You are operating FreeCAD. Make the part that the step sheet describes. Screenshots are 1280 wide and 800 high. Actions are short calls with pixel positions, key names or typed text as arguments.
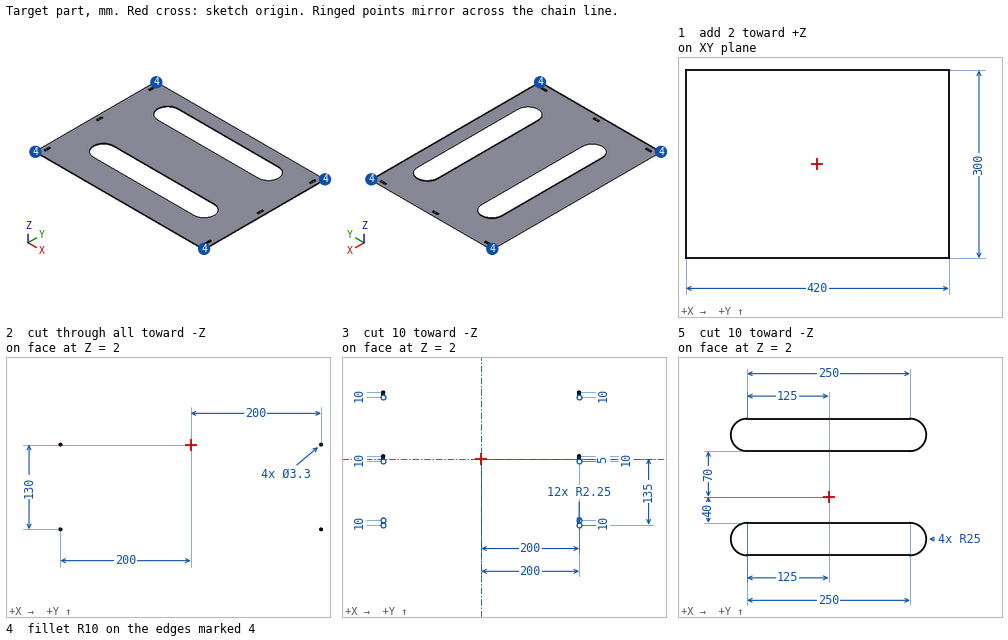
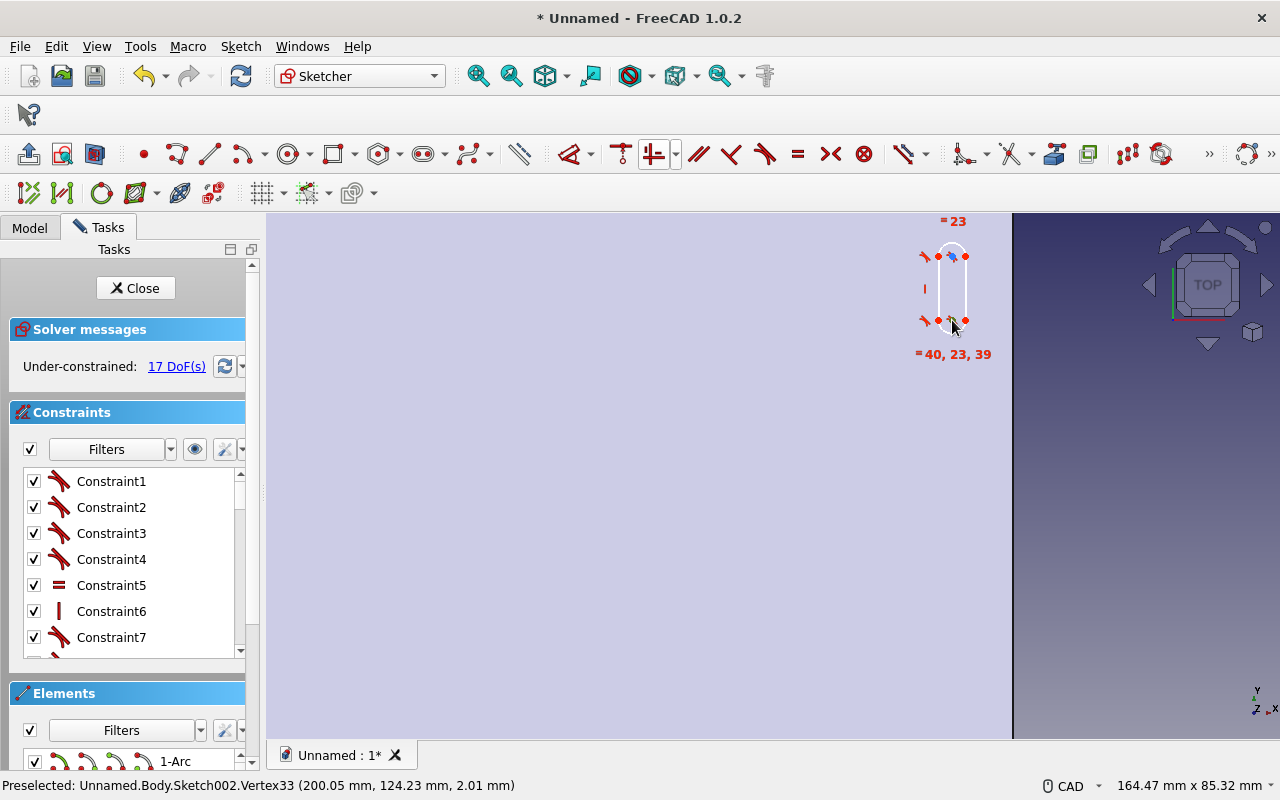
scroll(954, 322, down, 8)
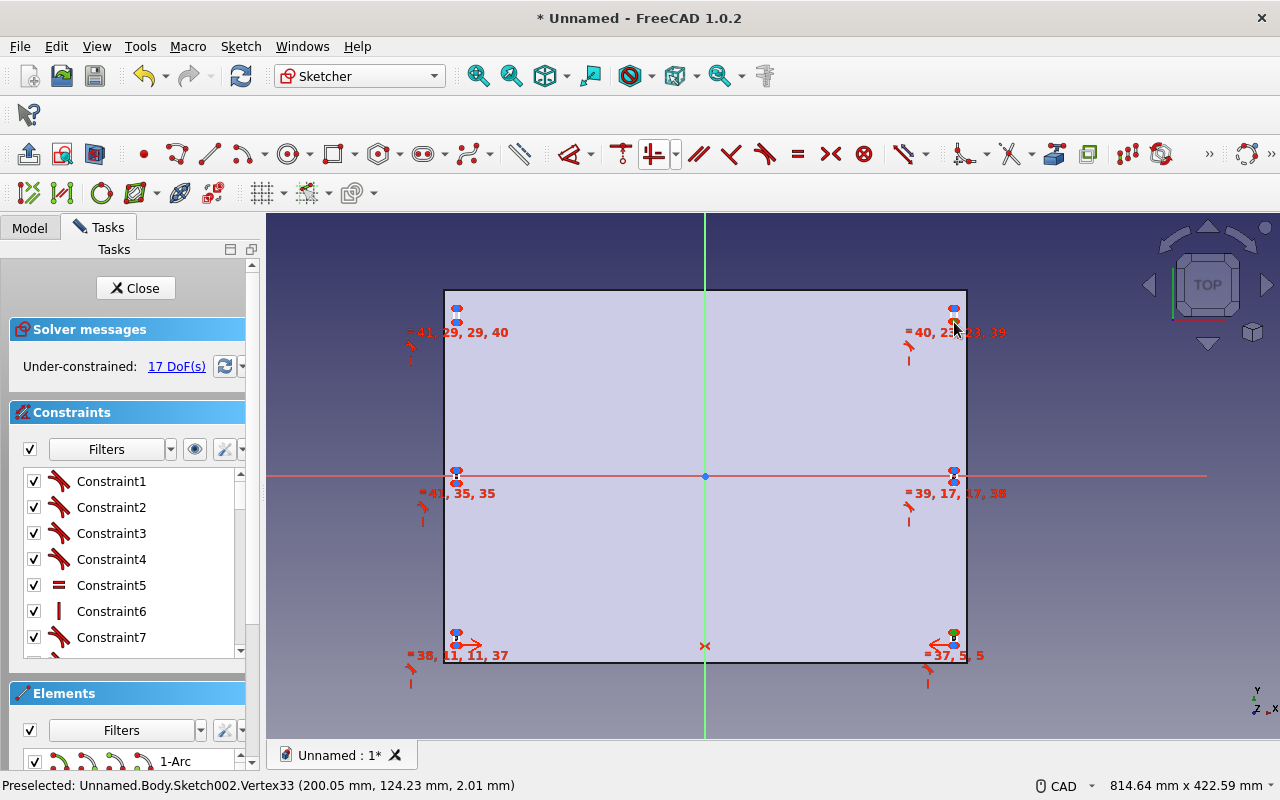
click(353, 476)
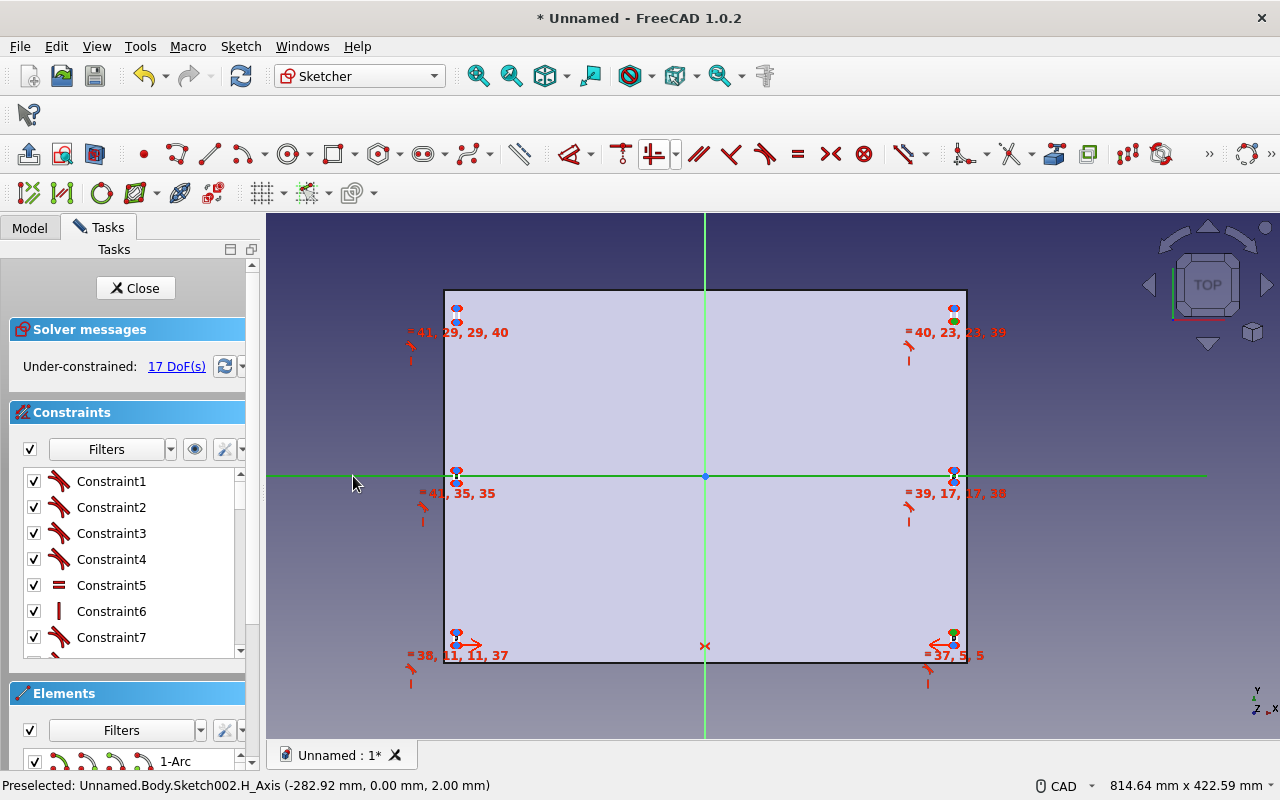
click(831, 154)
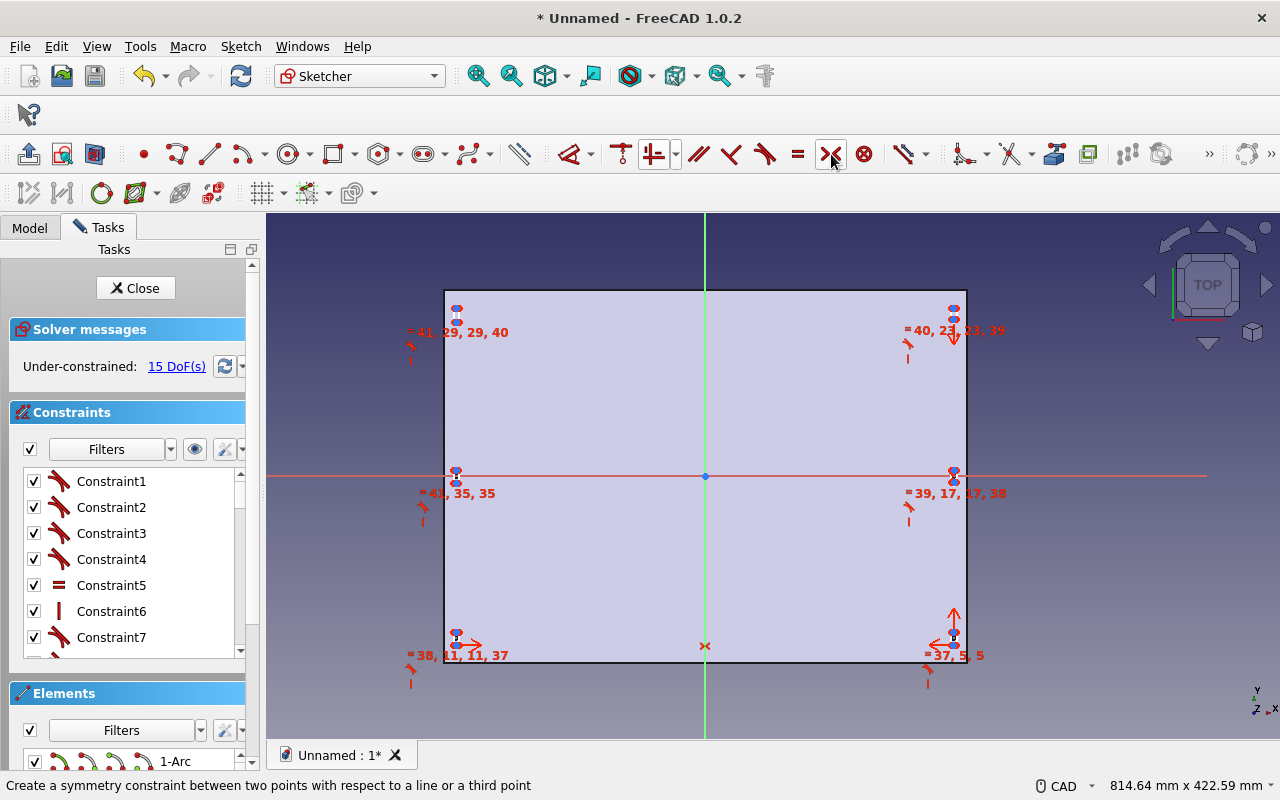
scroll(456, 633, up, 8)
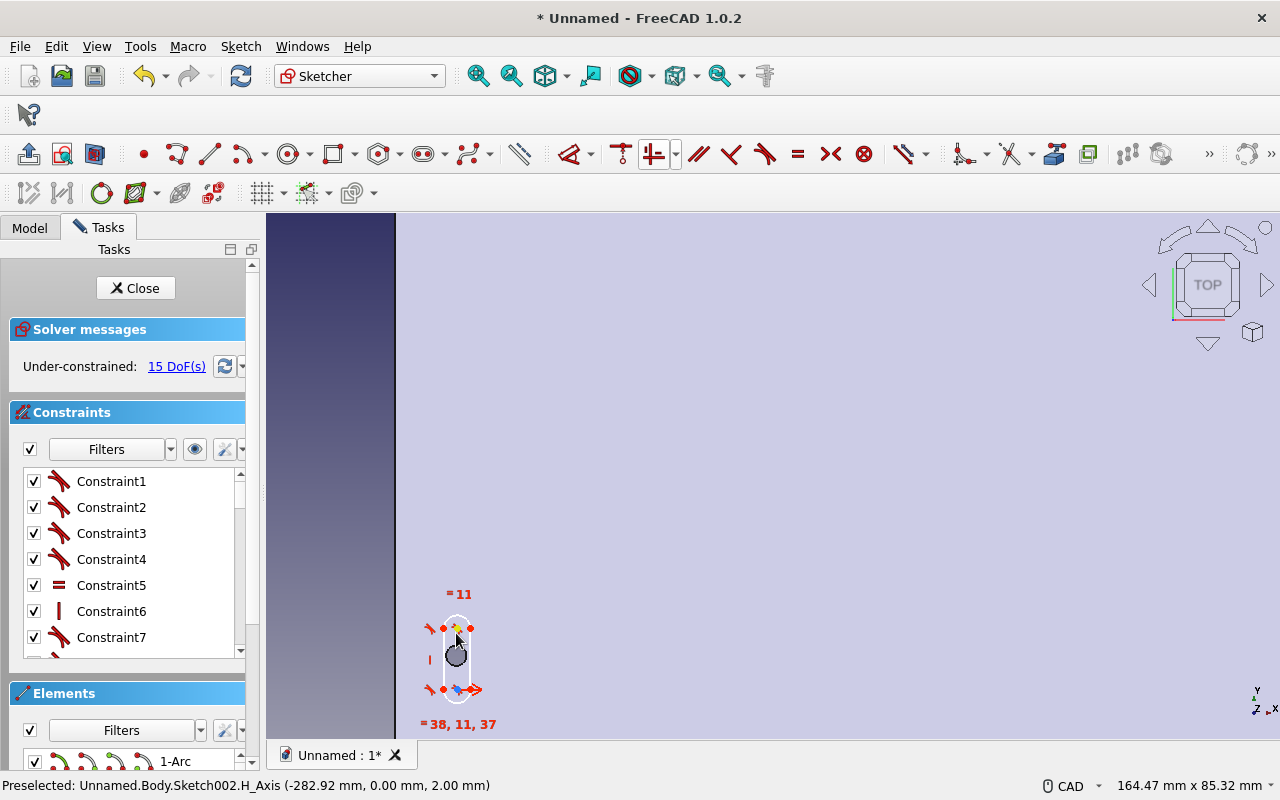
click(457, 629)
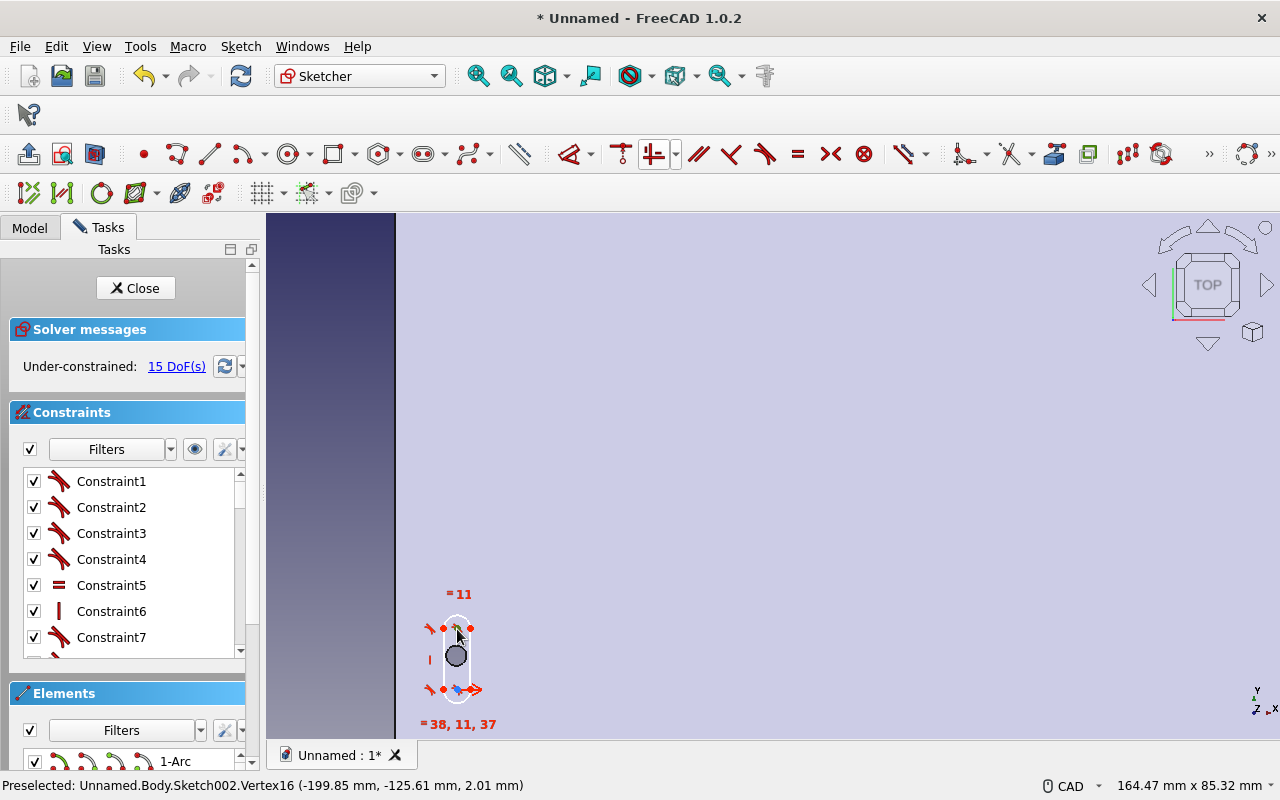
scroll(455, 633, down, 8)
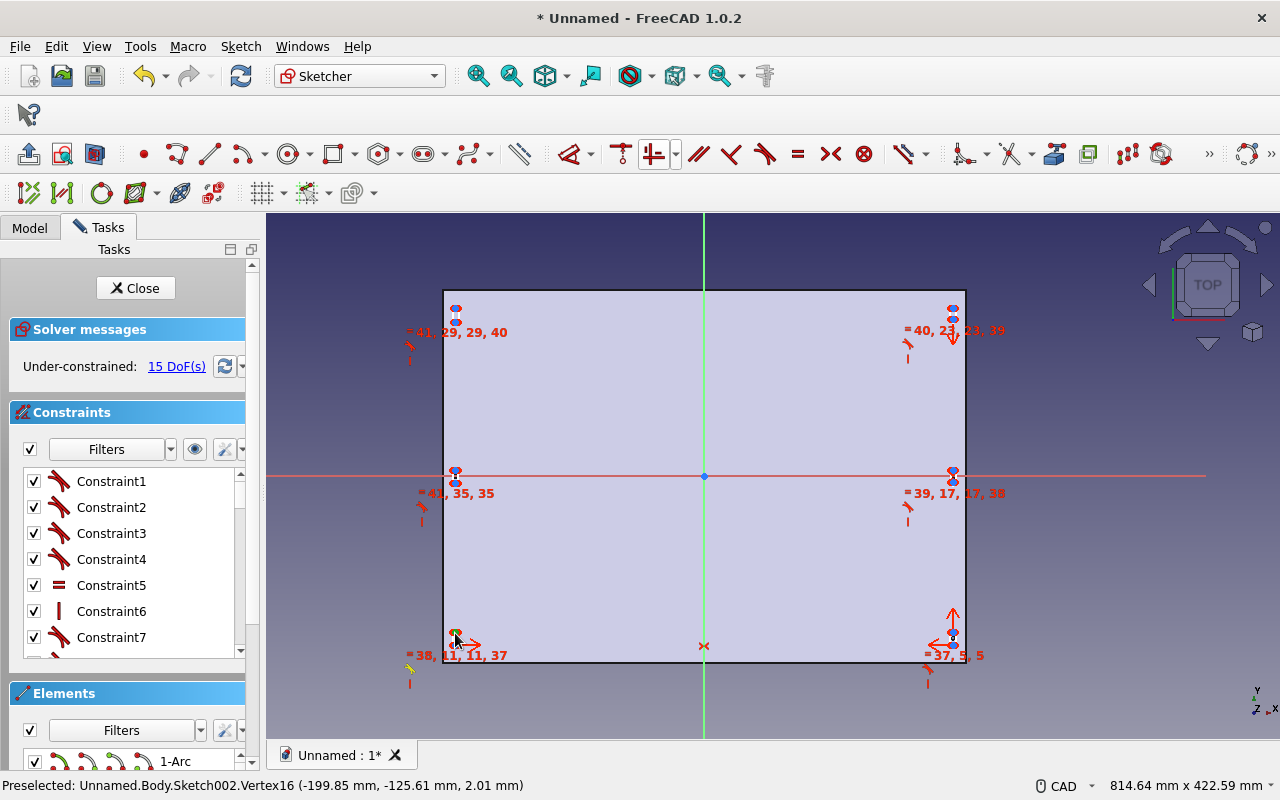
scroll(456, 322, up, 8)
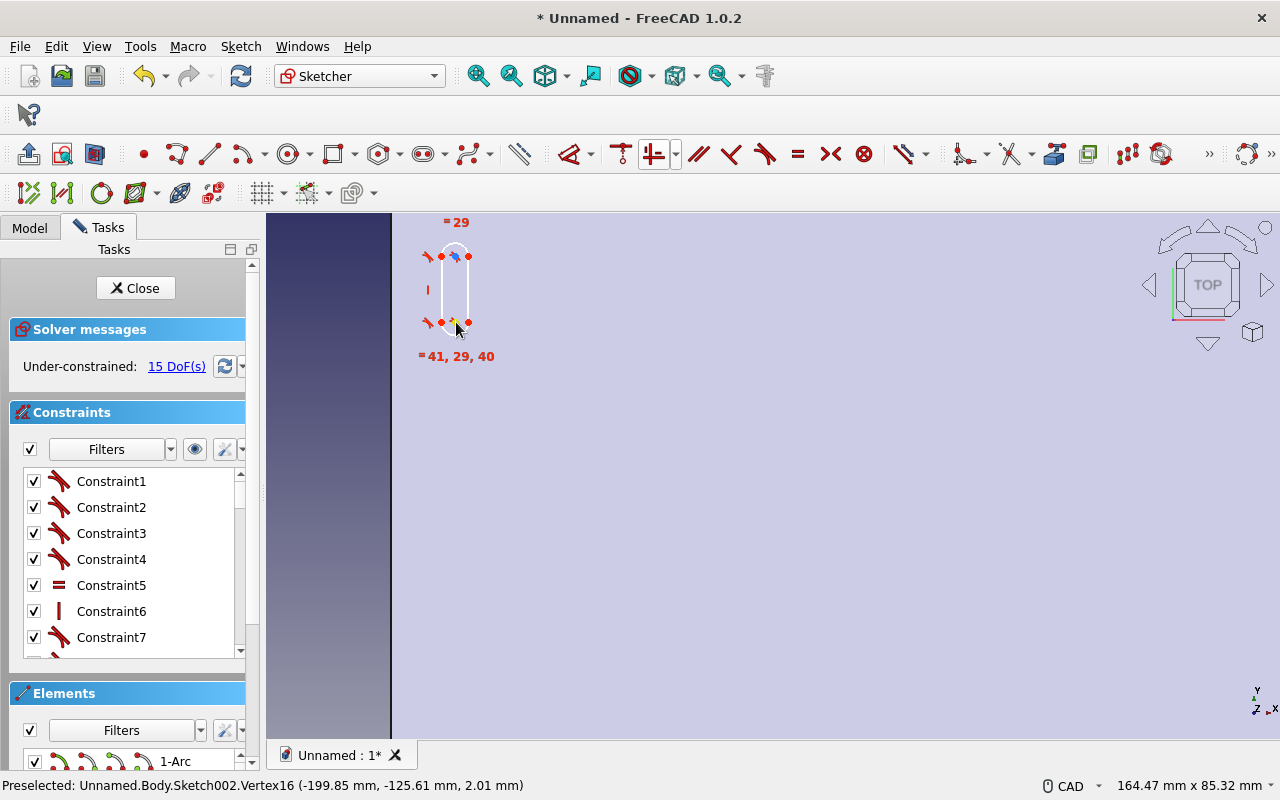
click(455, 322)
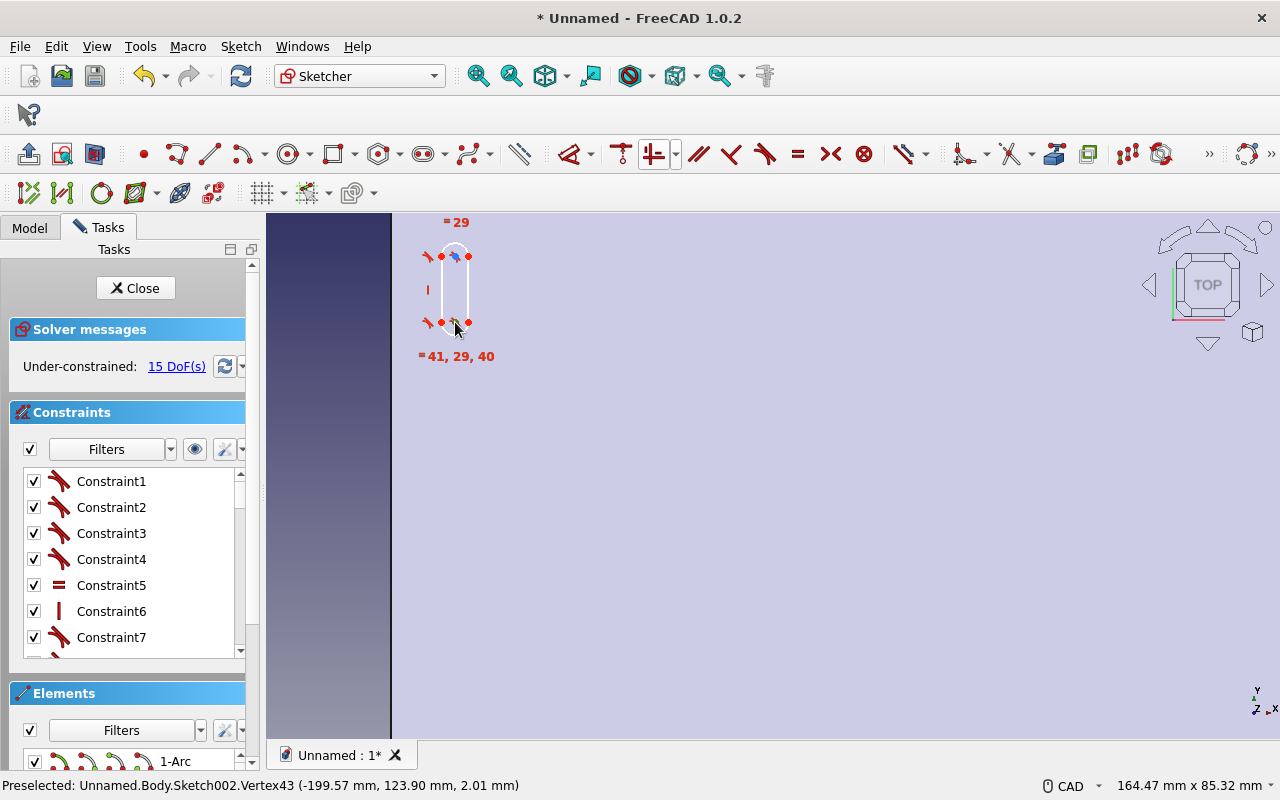
scroll(456, 322, down, 8)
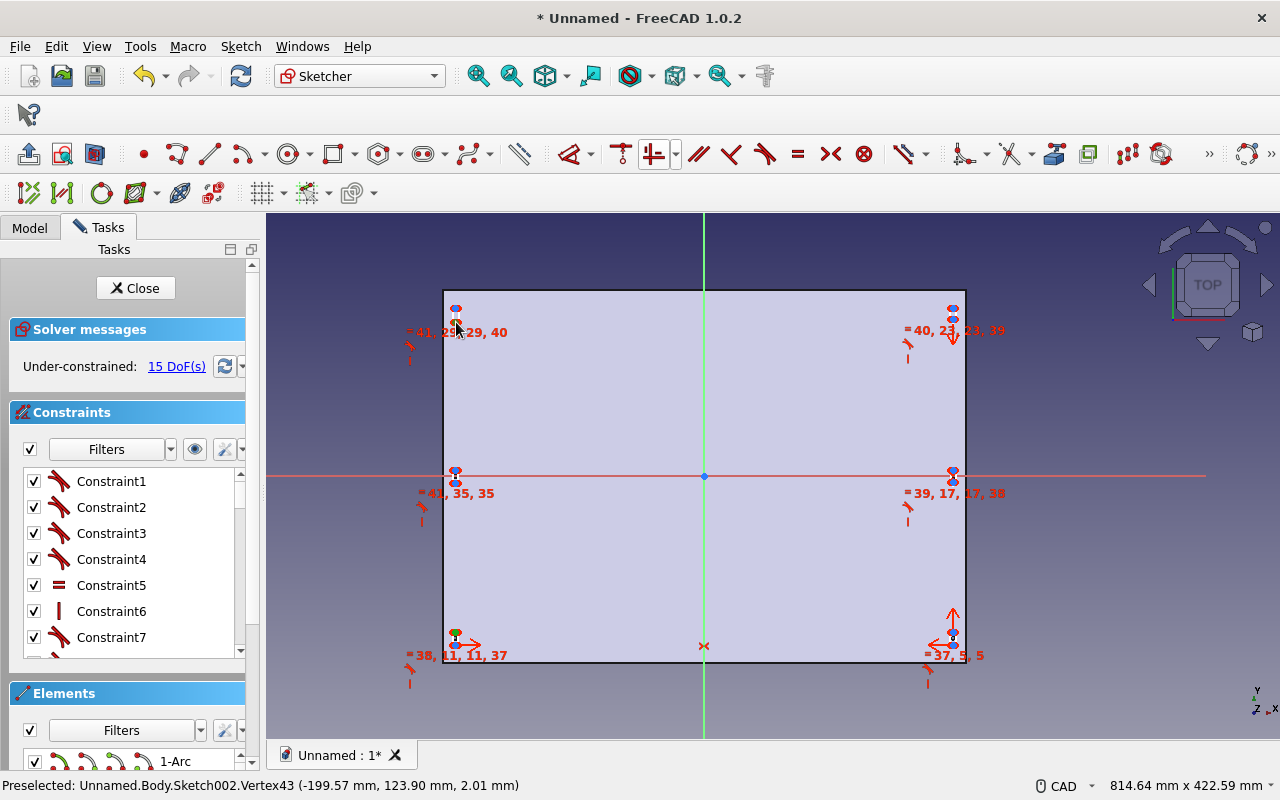
click(353, 476)